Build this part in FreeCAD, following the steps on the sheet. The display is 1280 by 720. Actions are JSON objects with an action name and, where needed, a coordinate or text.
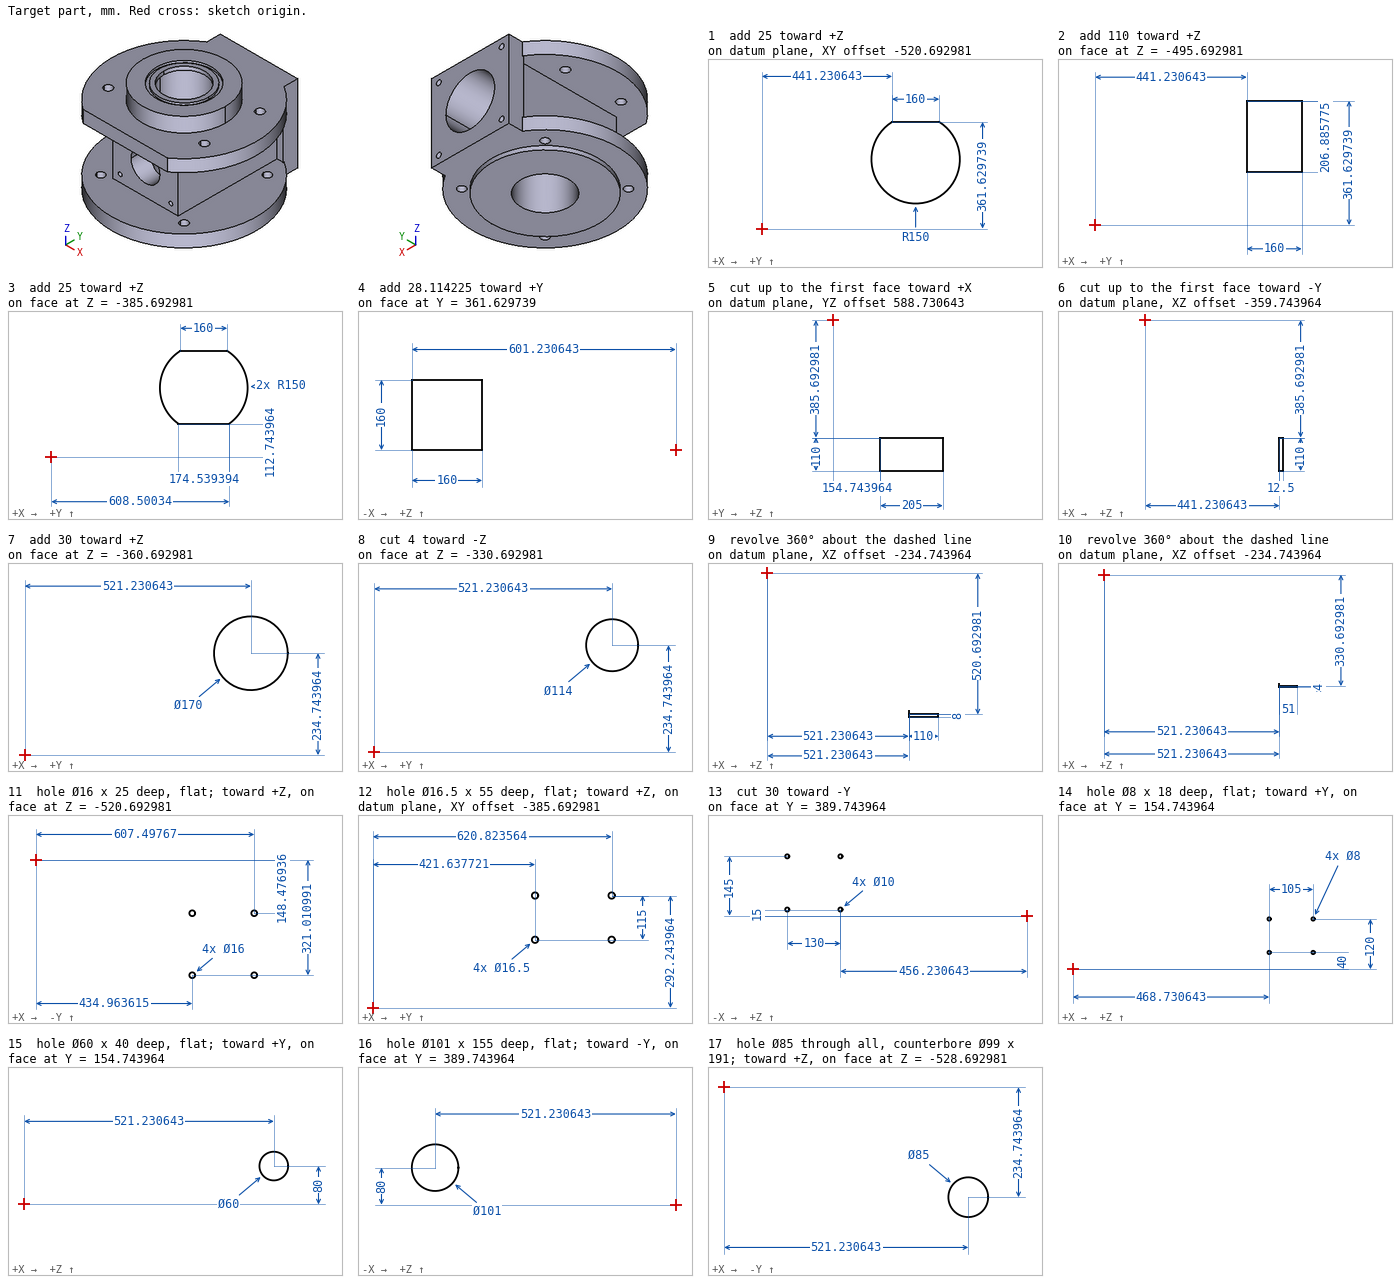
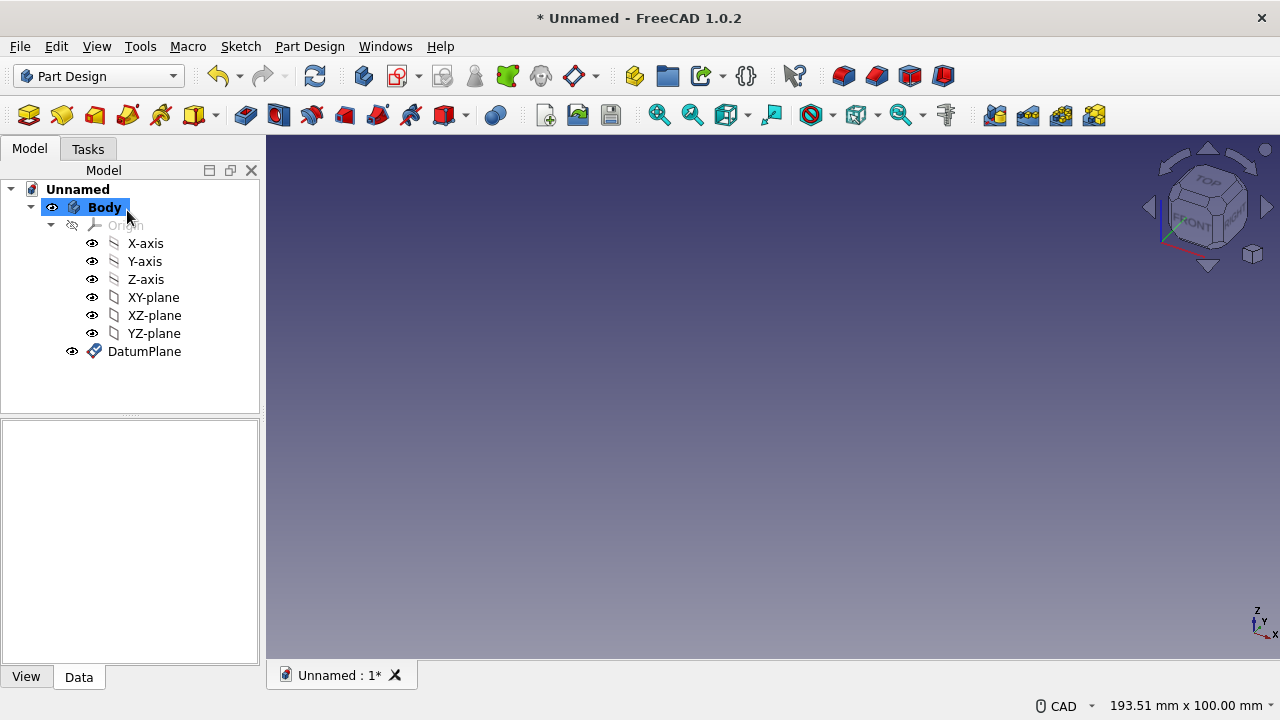
{"action": "left_click", "coordinate": [117, 351]}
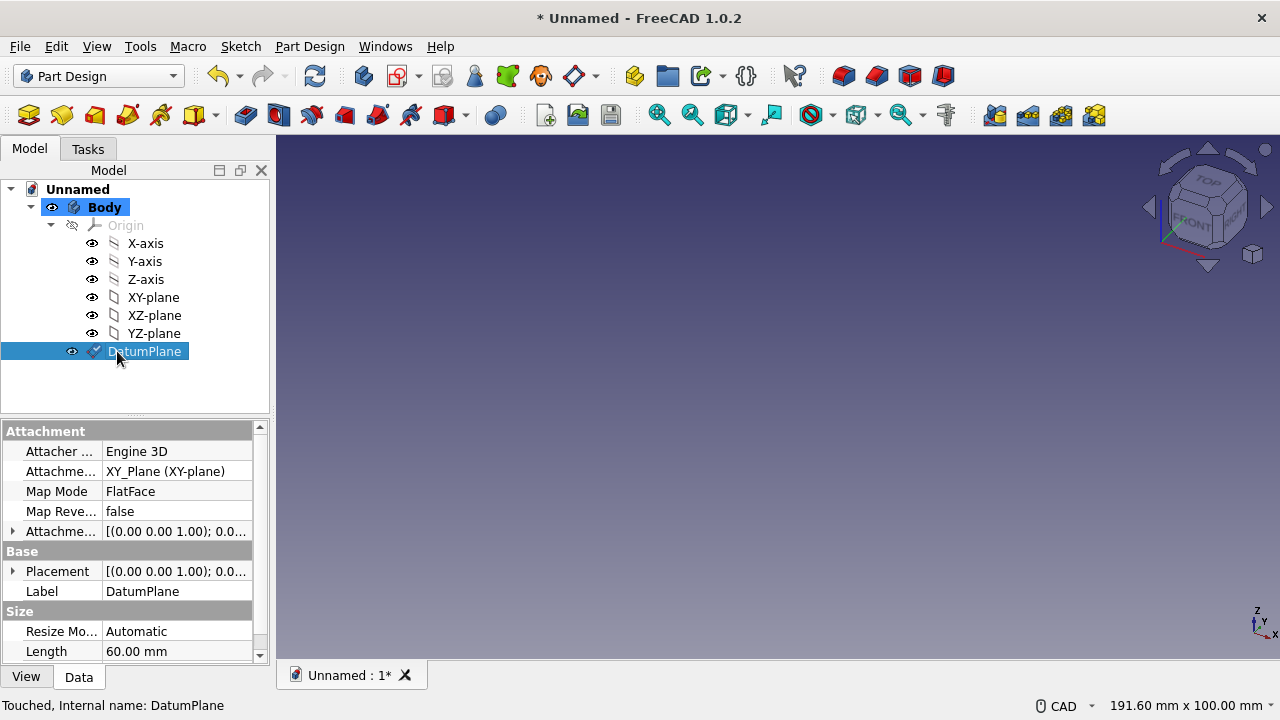
{"action": "left_click", "coordinate": [396, 76]}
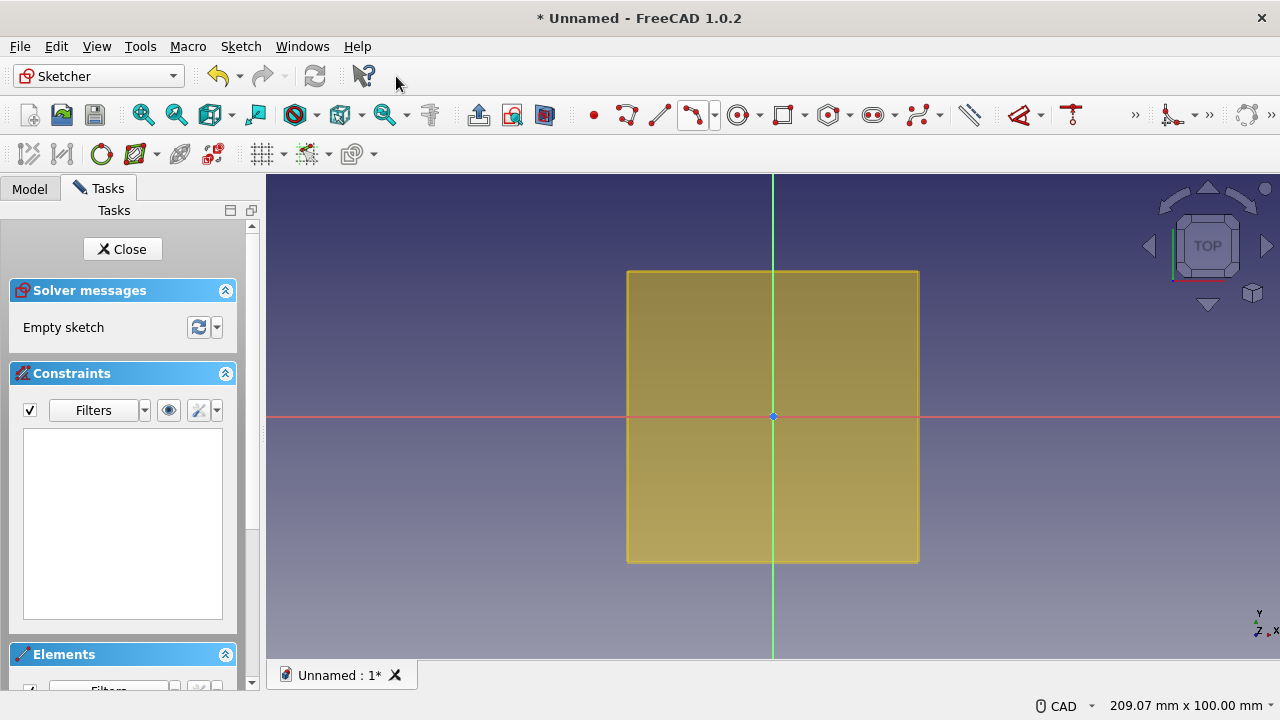
{"action": "scroll", "coordinate": [402, 590], "scroll_direction": "down", "scroll_amount": 9}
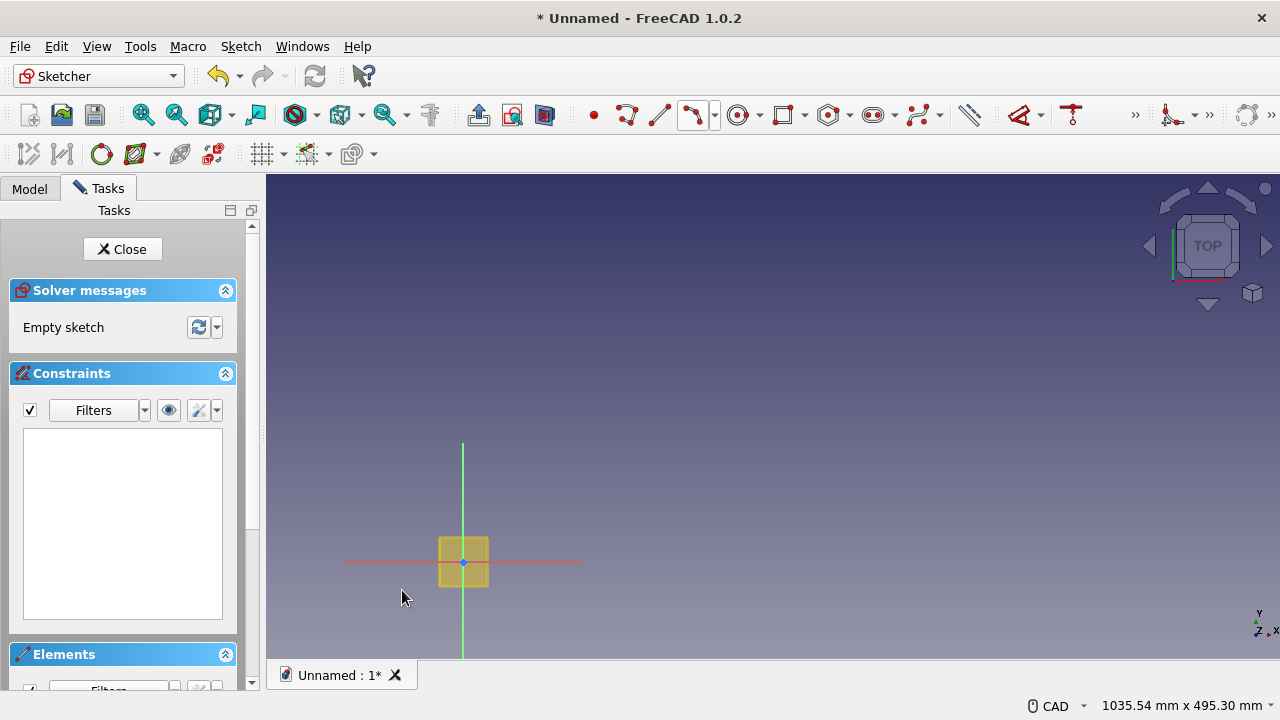
{"action": "left_click", "coordinate": [660, 116]}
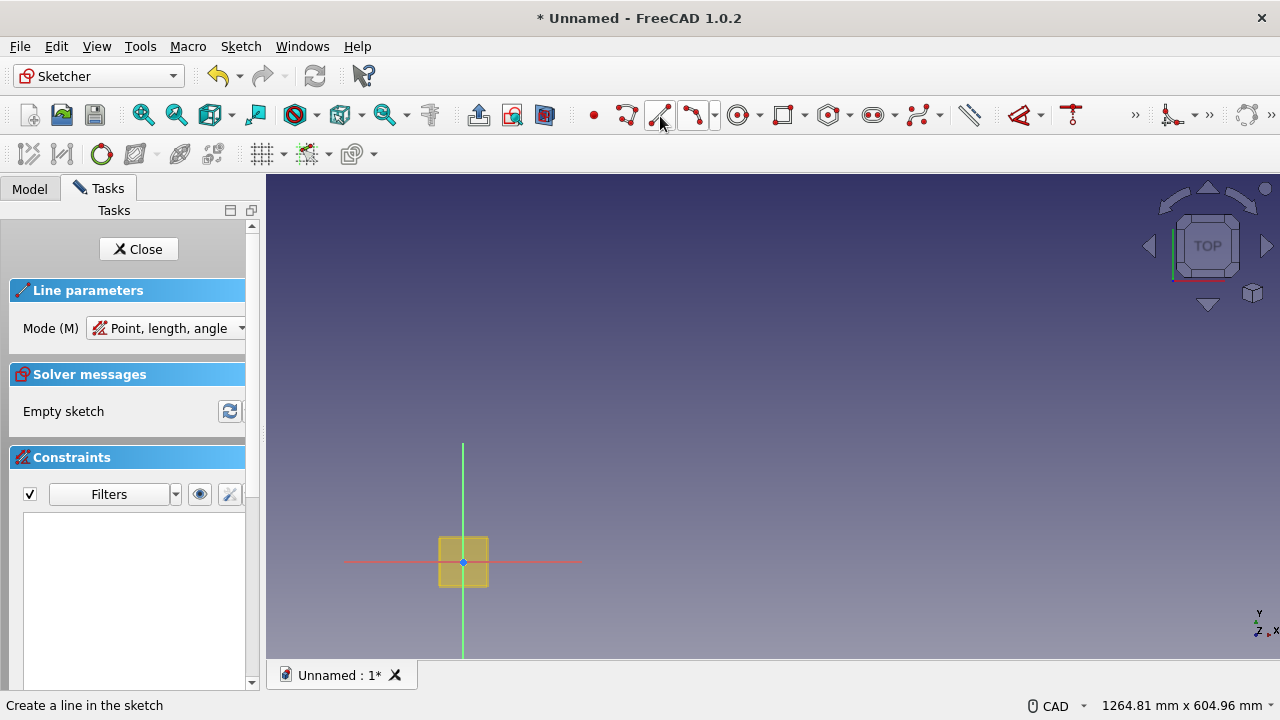
{"action": "left_click", "coordinate": [817, 272]}
{"action": "left_click", "coordinate": [945, 272]}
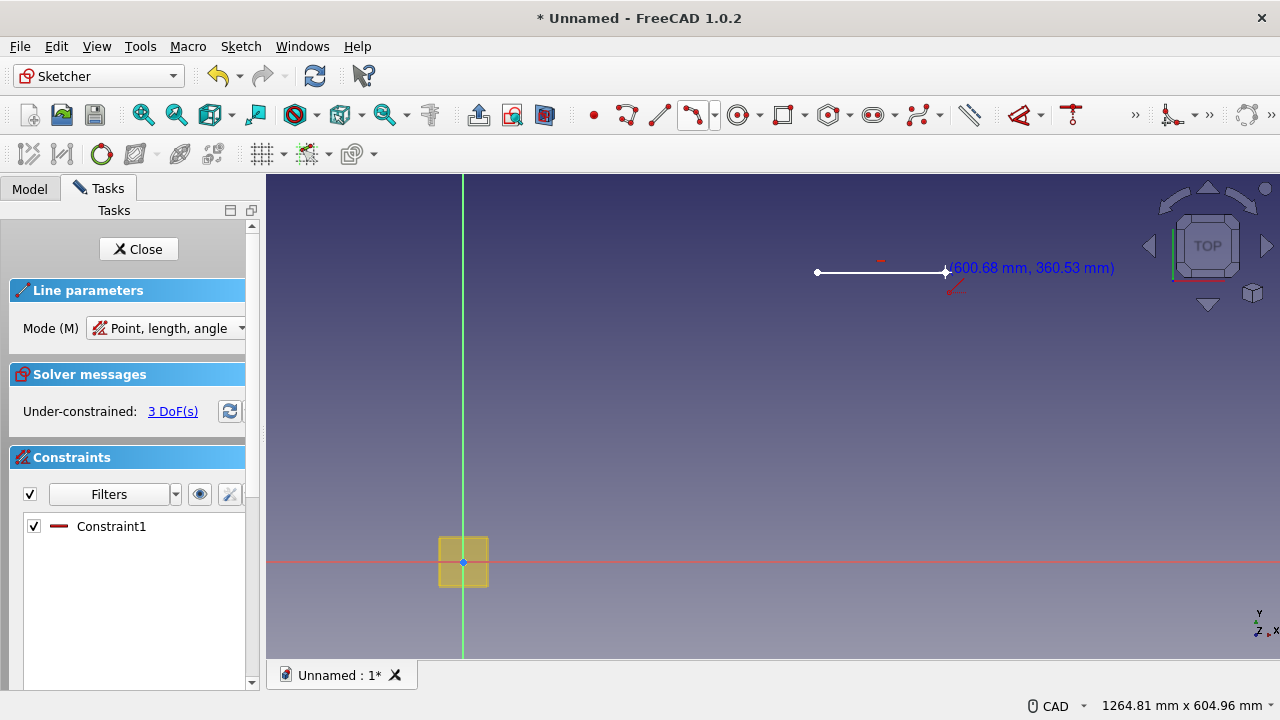
{"action": "left_click", "coordinate": [692, 116]}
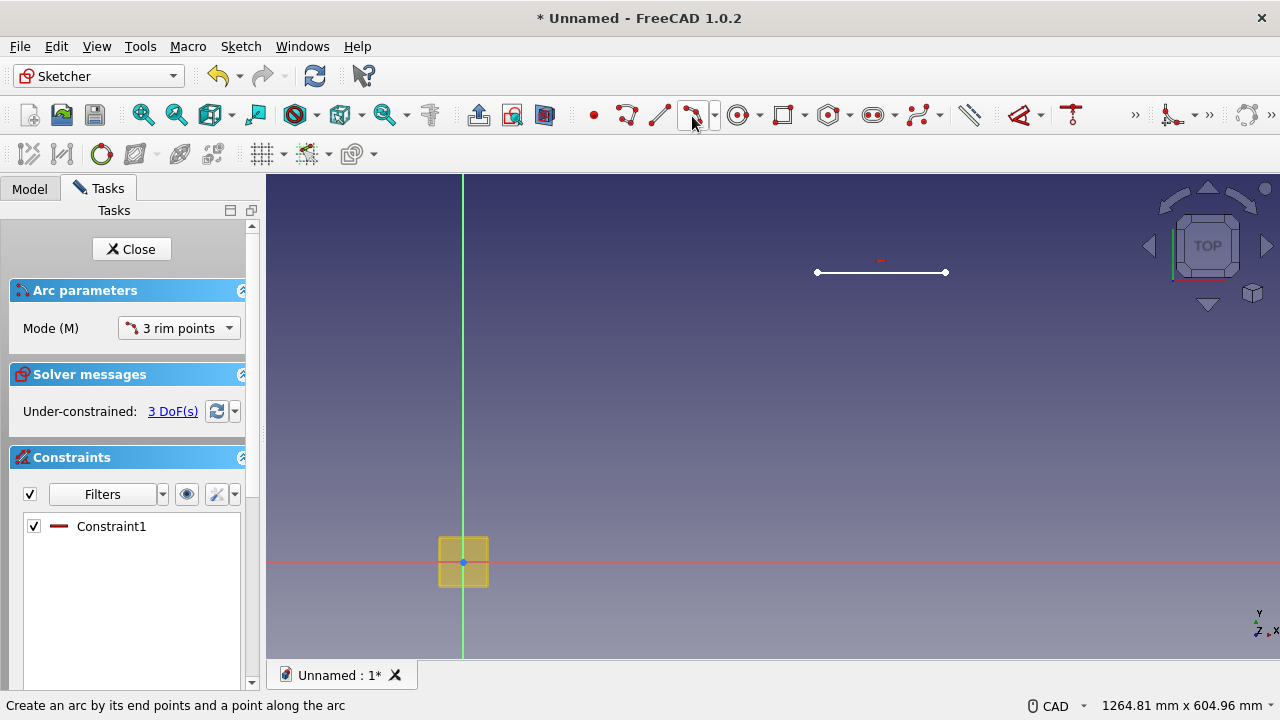
{"action": "left_click", "coordinate": [945, 273]}
{"action": "left_click", "coordinate": [817, 273]}
{"action": "left_click", "coordinate": [881, 494]}
{"action": "key", "text": "Escape"}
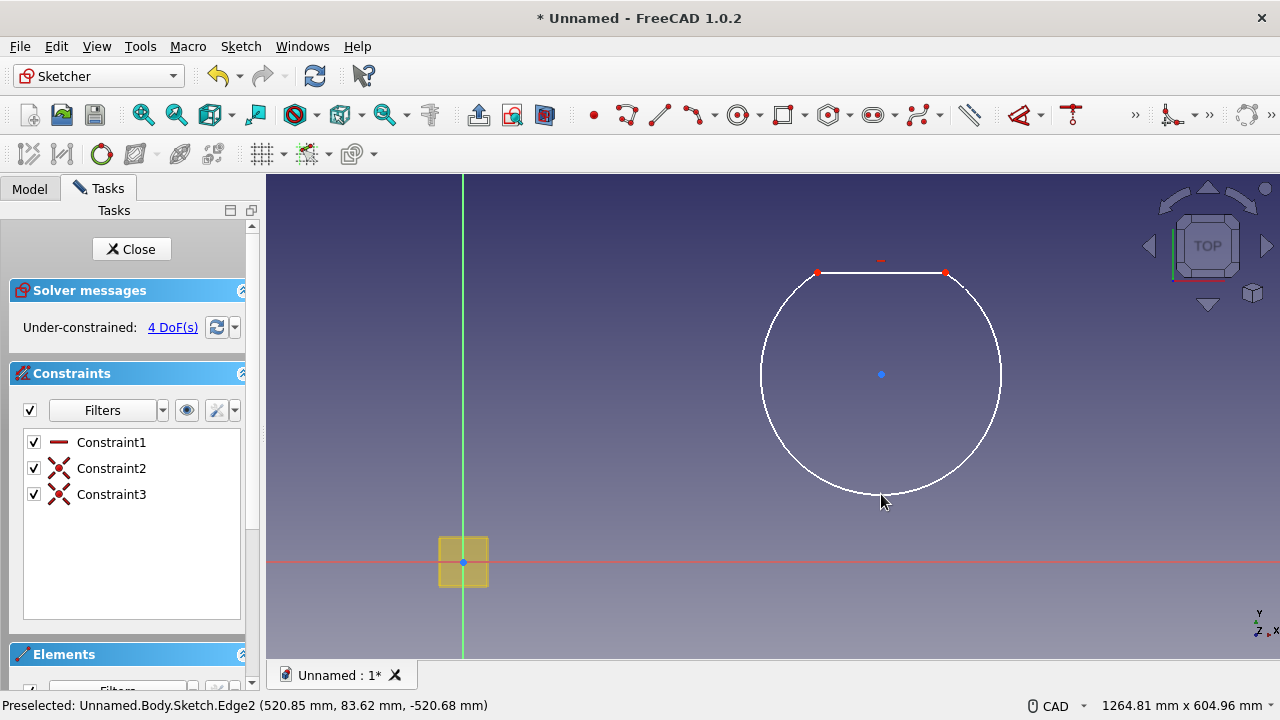
{"action": "left_click", "coordinate": [778, 436]}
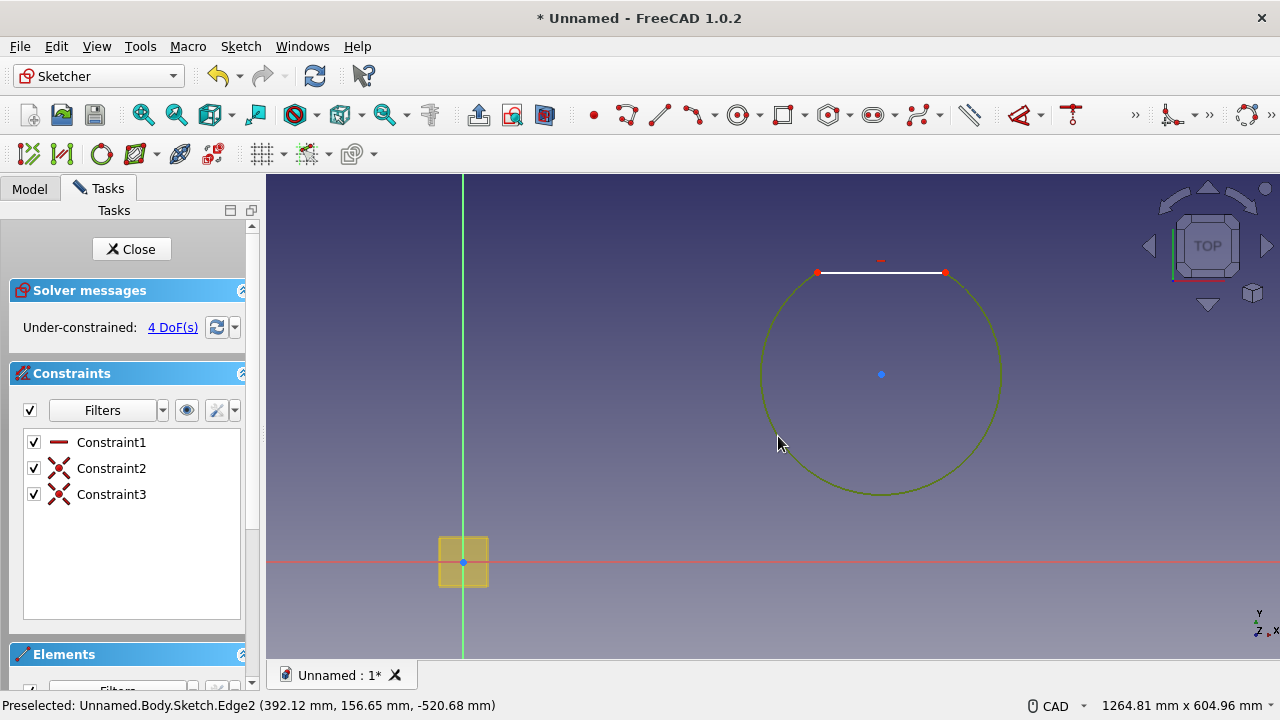
{"action": "key", "text": "k r"}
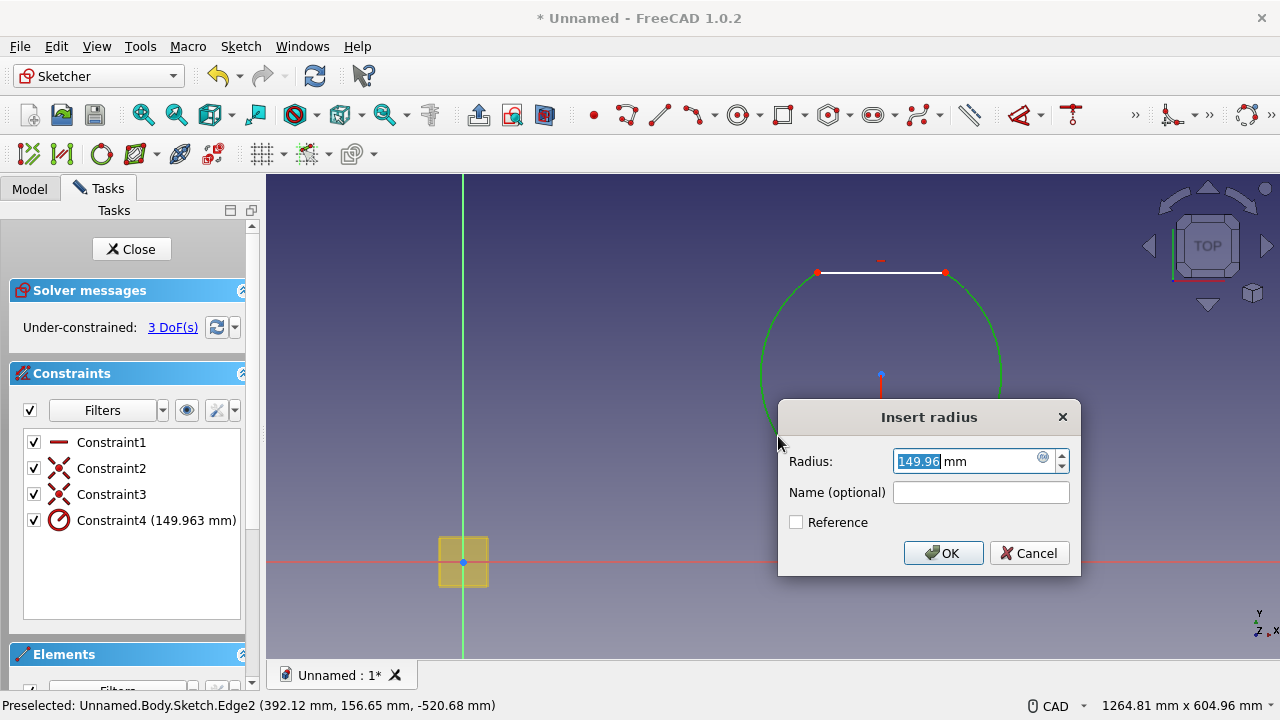
{"action": "type", "text": "150"}
{"action": "key", "text": "Return"}